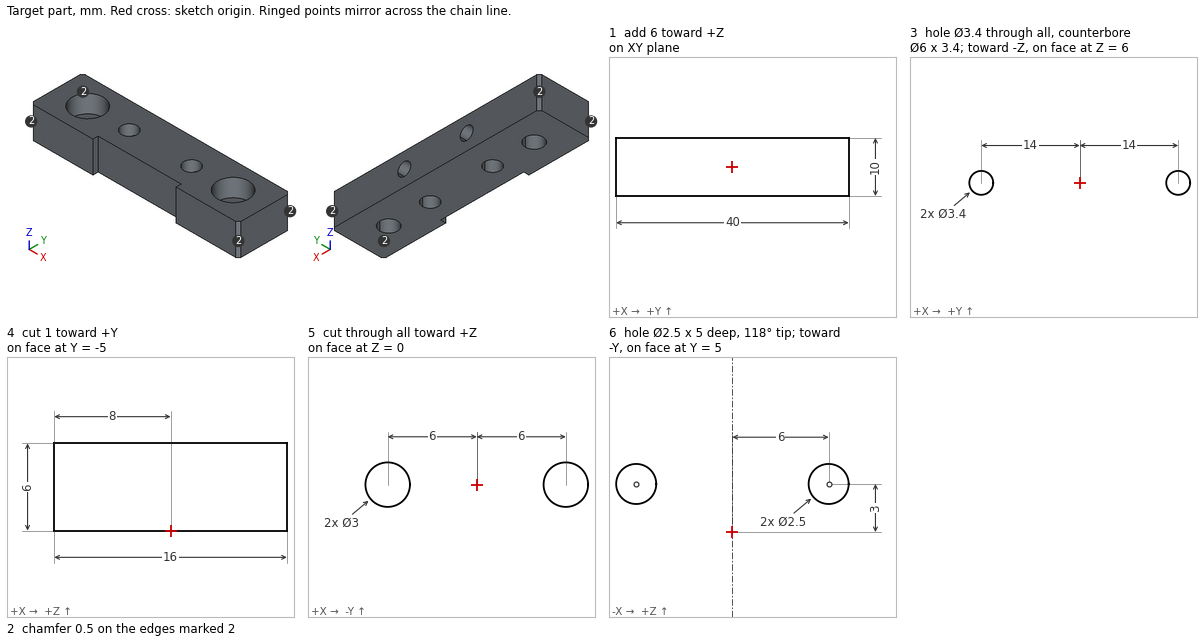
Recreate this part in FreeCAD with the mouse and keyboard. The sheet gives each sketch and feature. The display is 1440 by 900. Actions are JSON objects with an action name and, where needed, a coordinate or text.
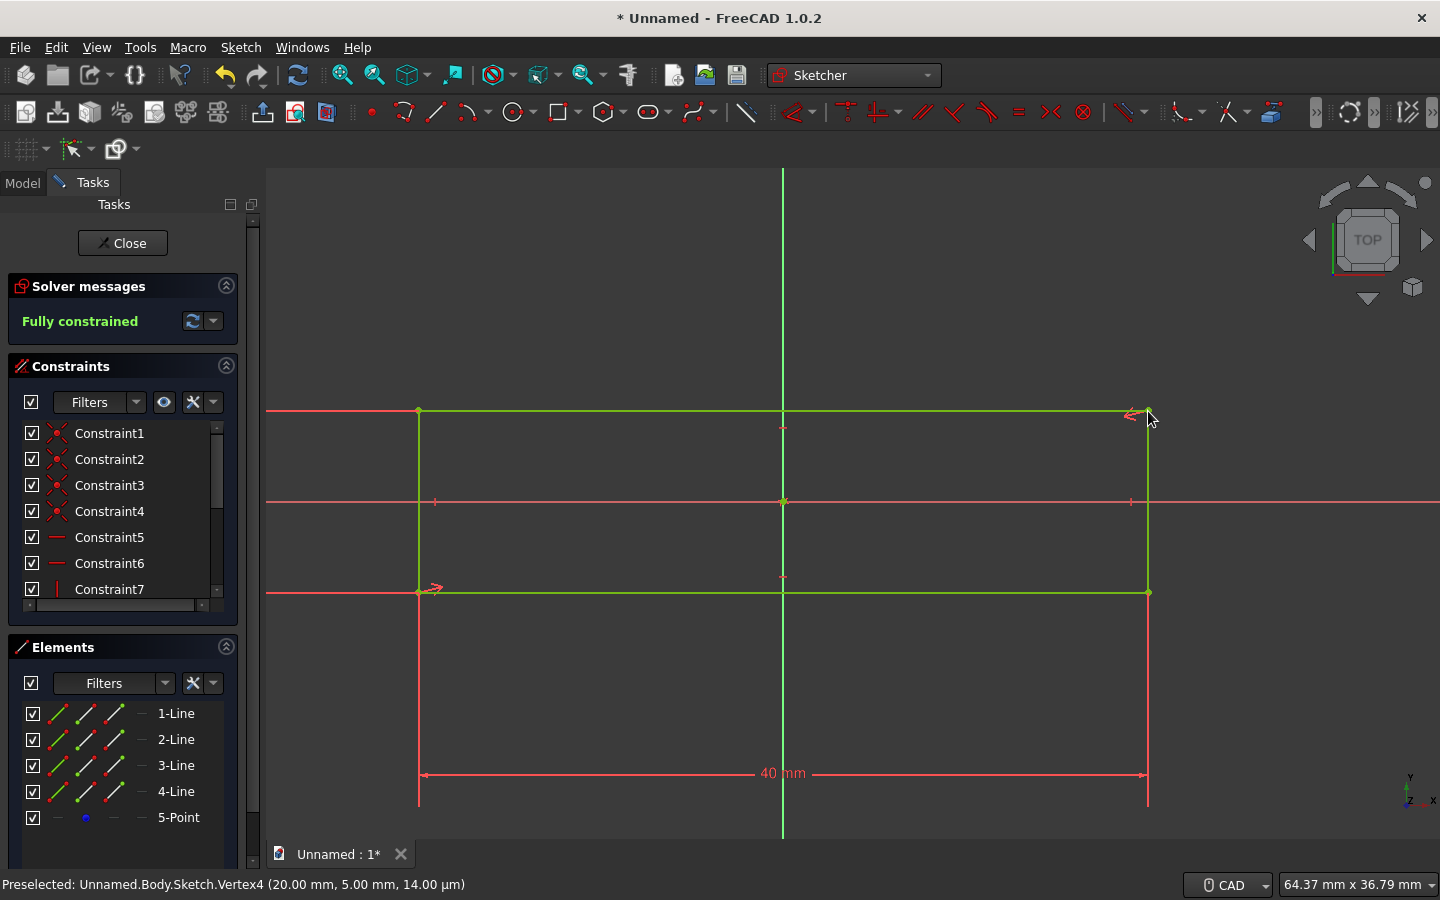
{"action": "left_click", "coordinate": [123, 243]}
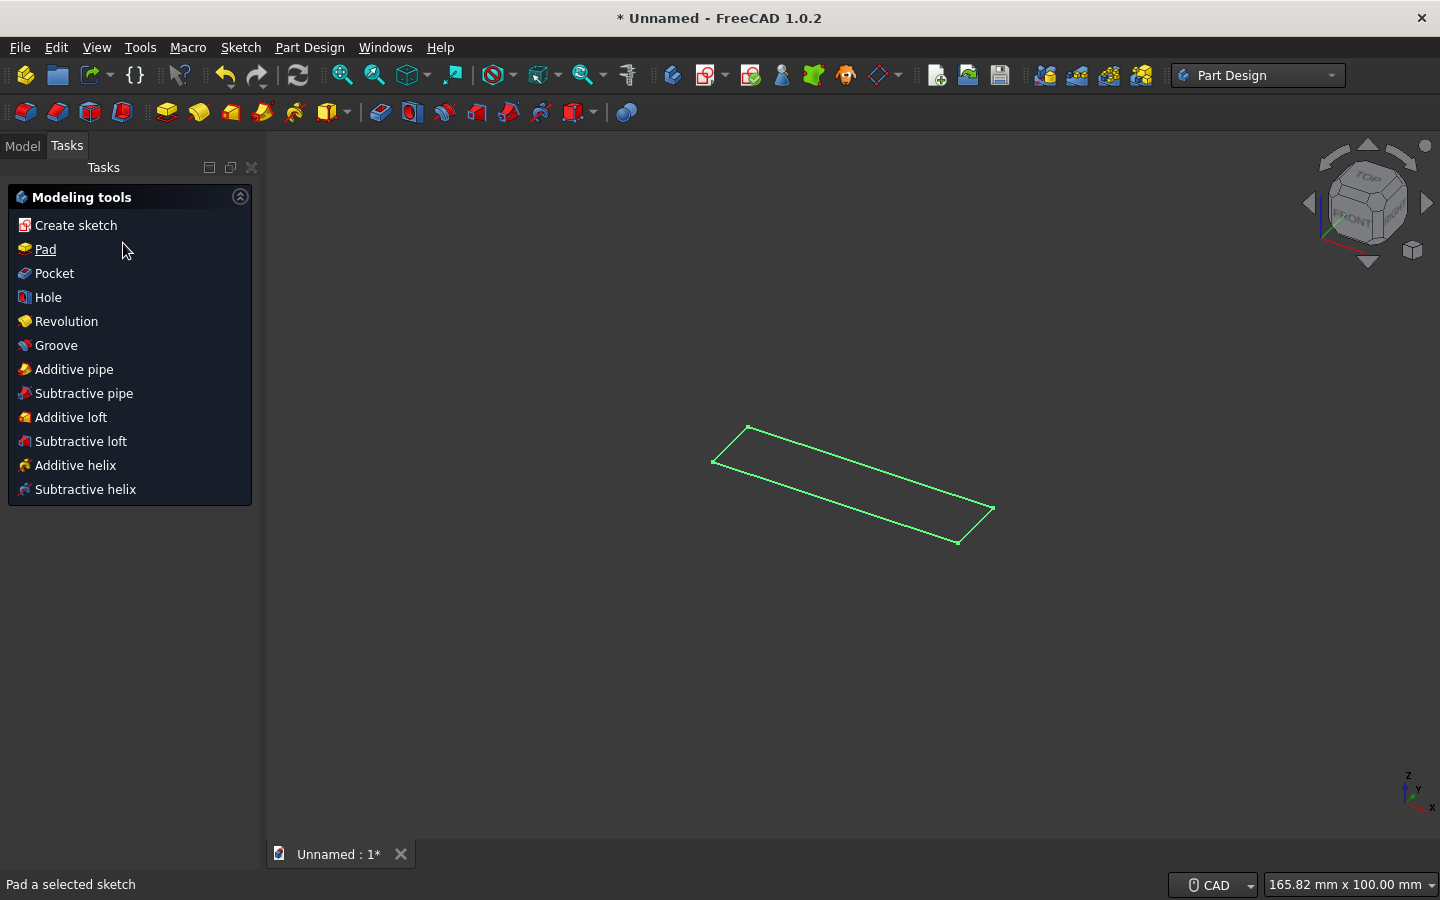
{"action": "left_click", "coordinate": [168, 112]}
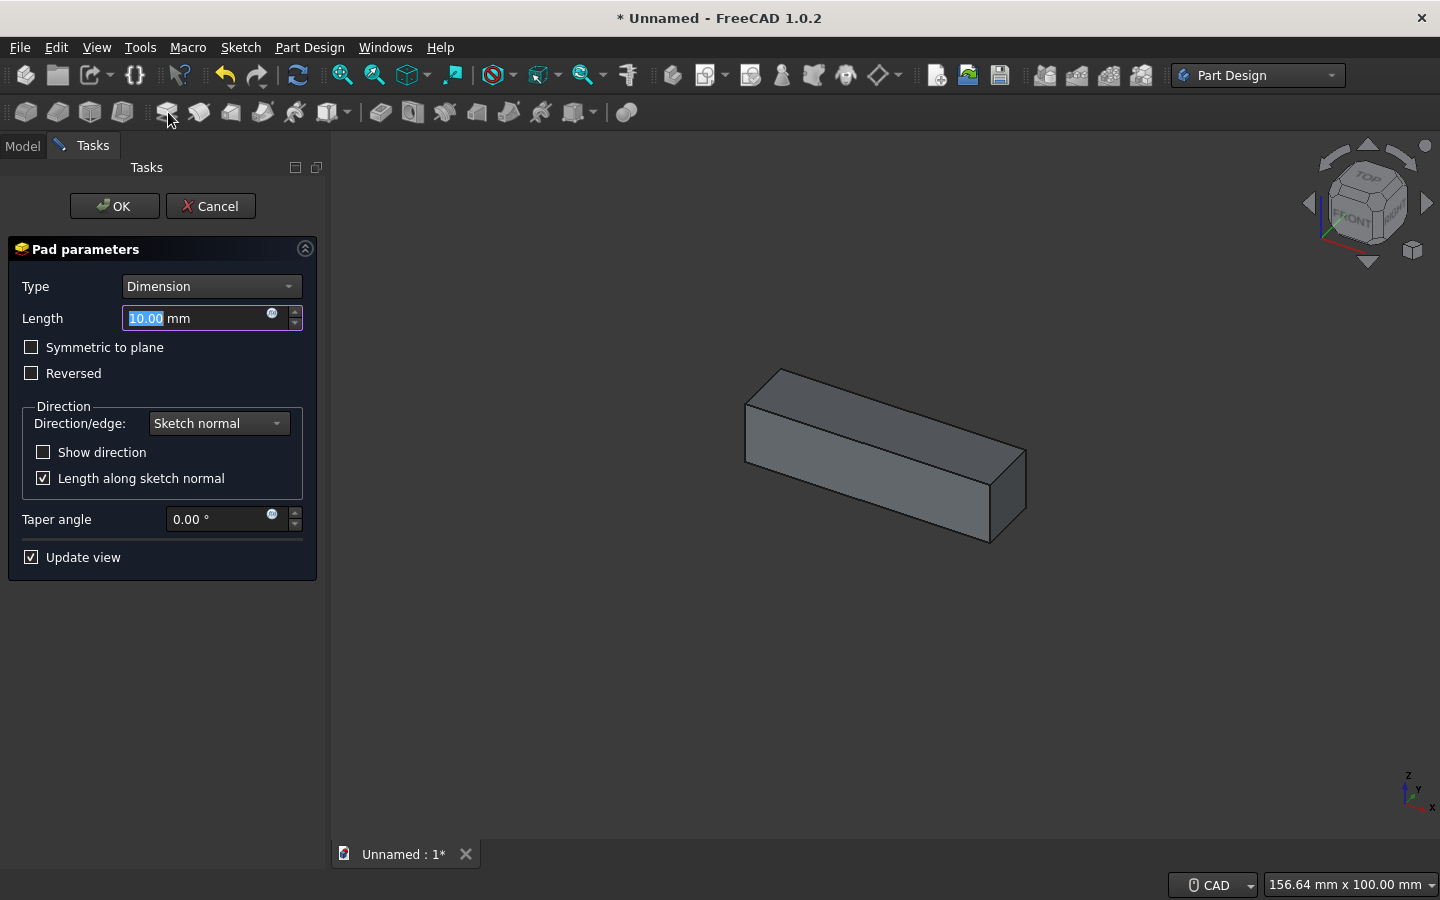
{"action": "type", "text": "6"}
{"action": "key", "text": "Tab"}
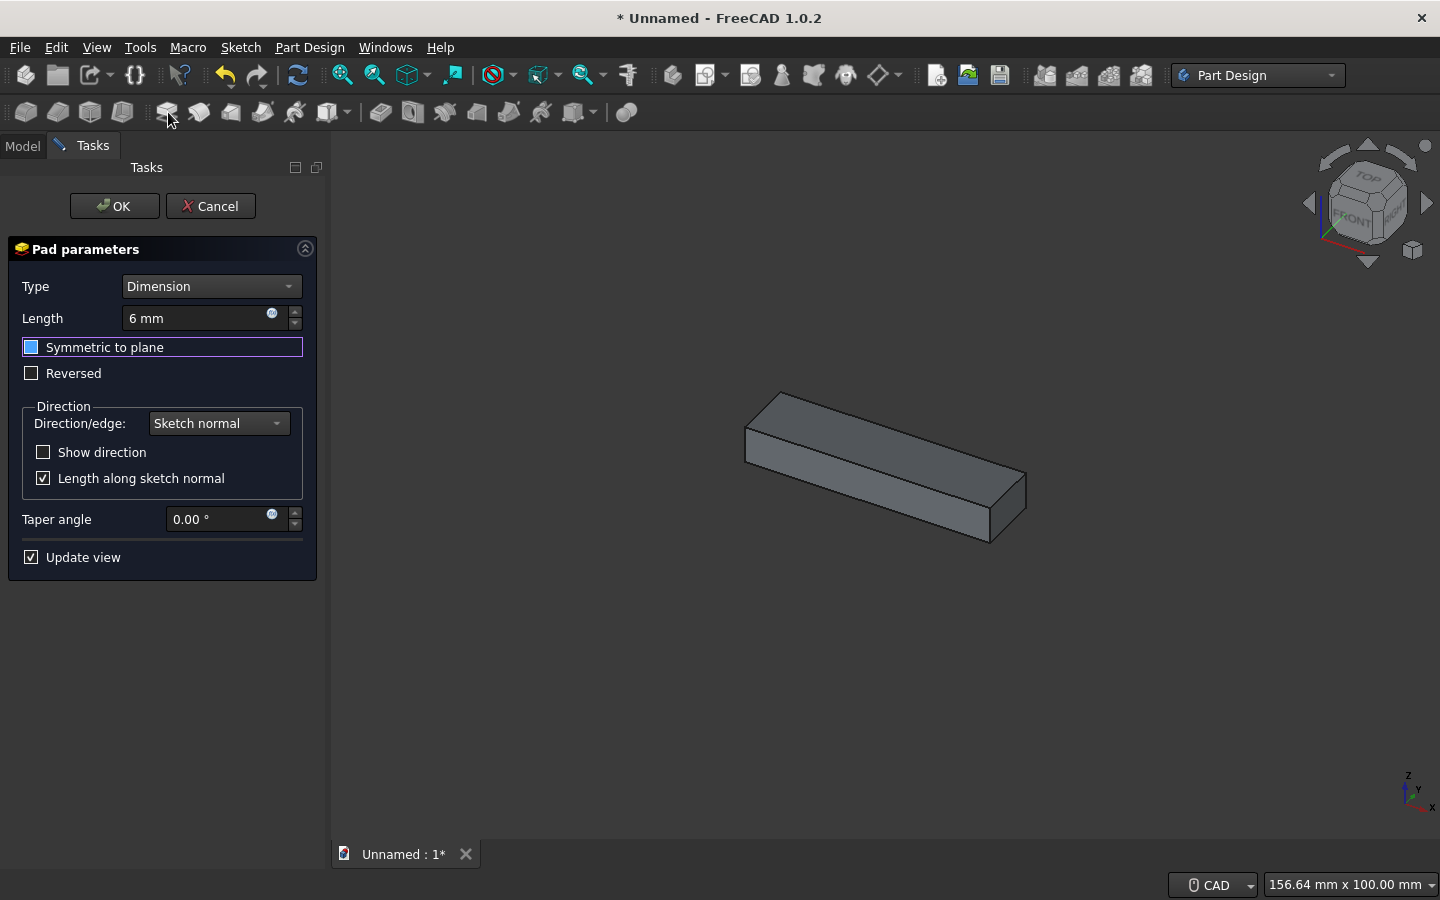
{"action": "left_click", "coordinate": [115, 206]}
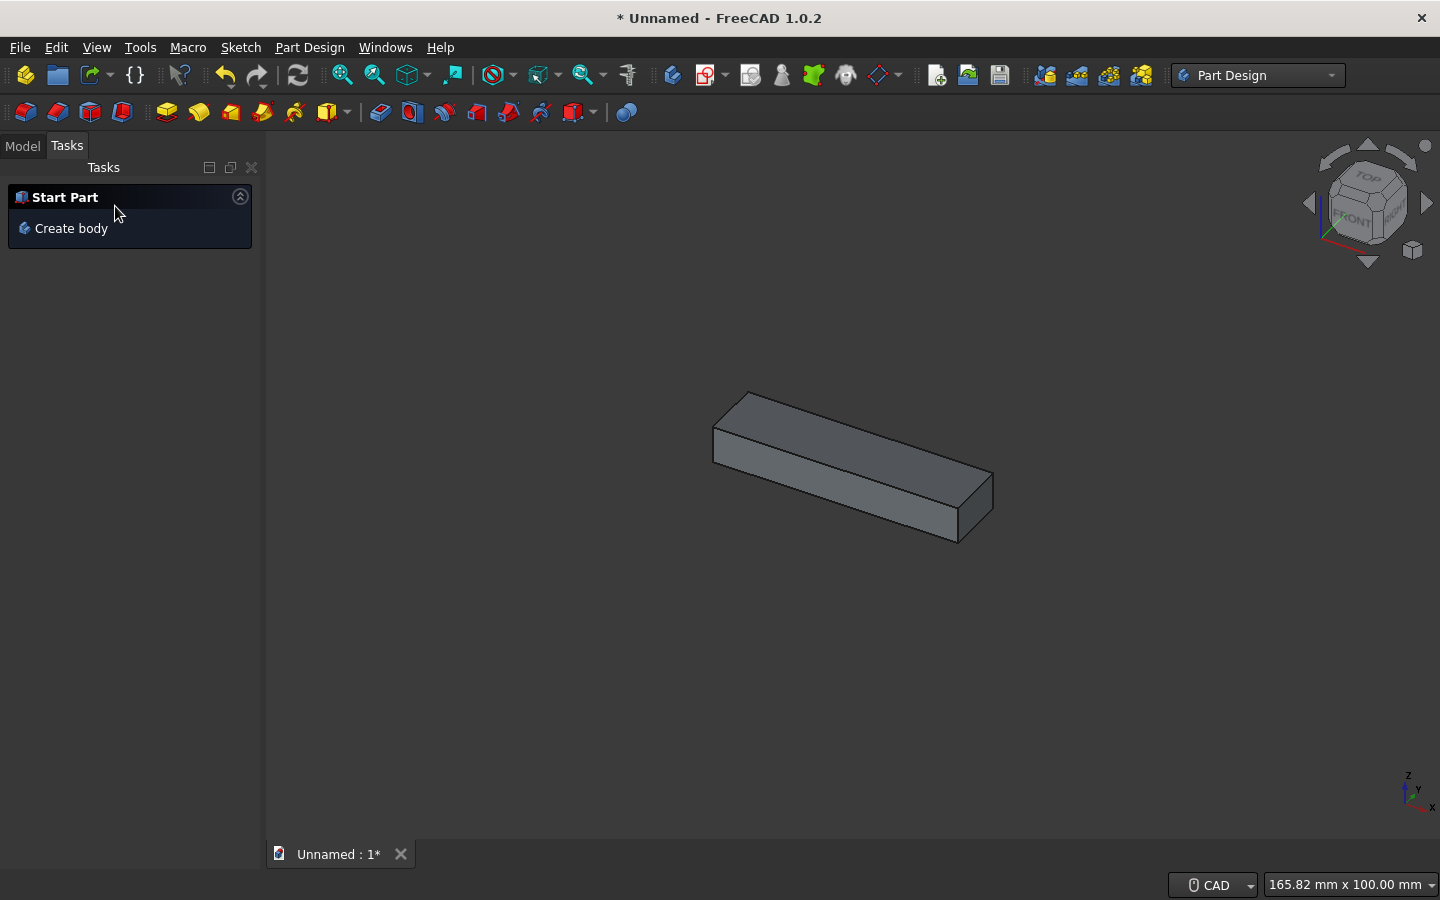
{"action": "left_click", "coordinate": [344, 76]}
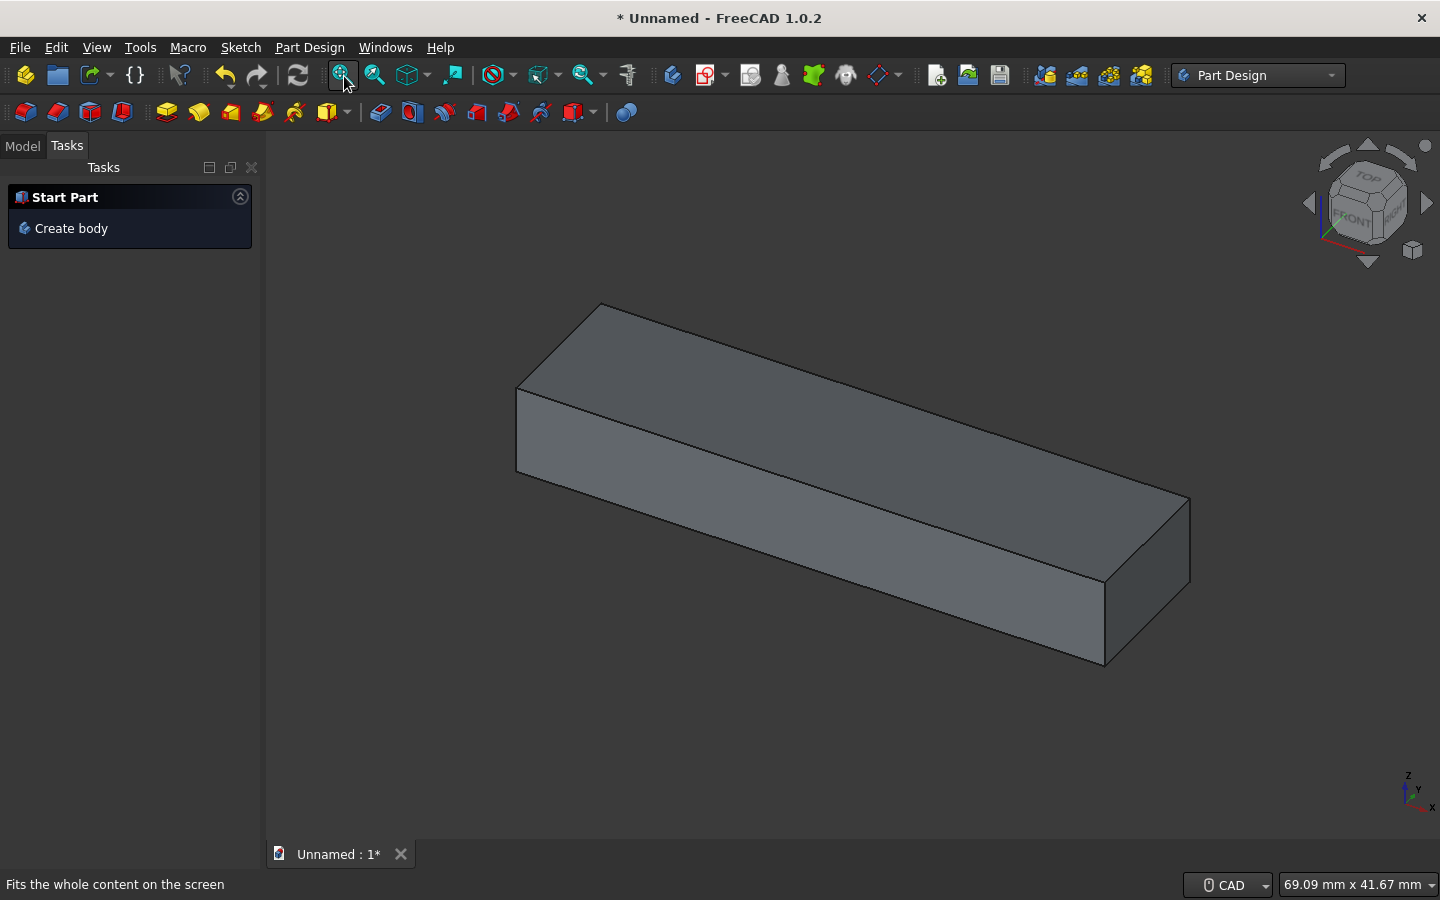
{"action": "left_click", "coordinate": [1105, 624]}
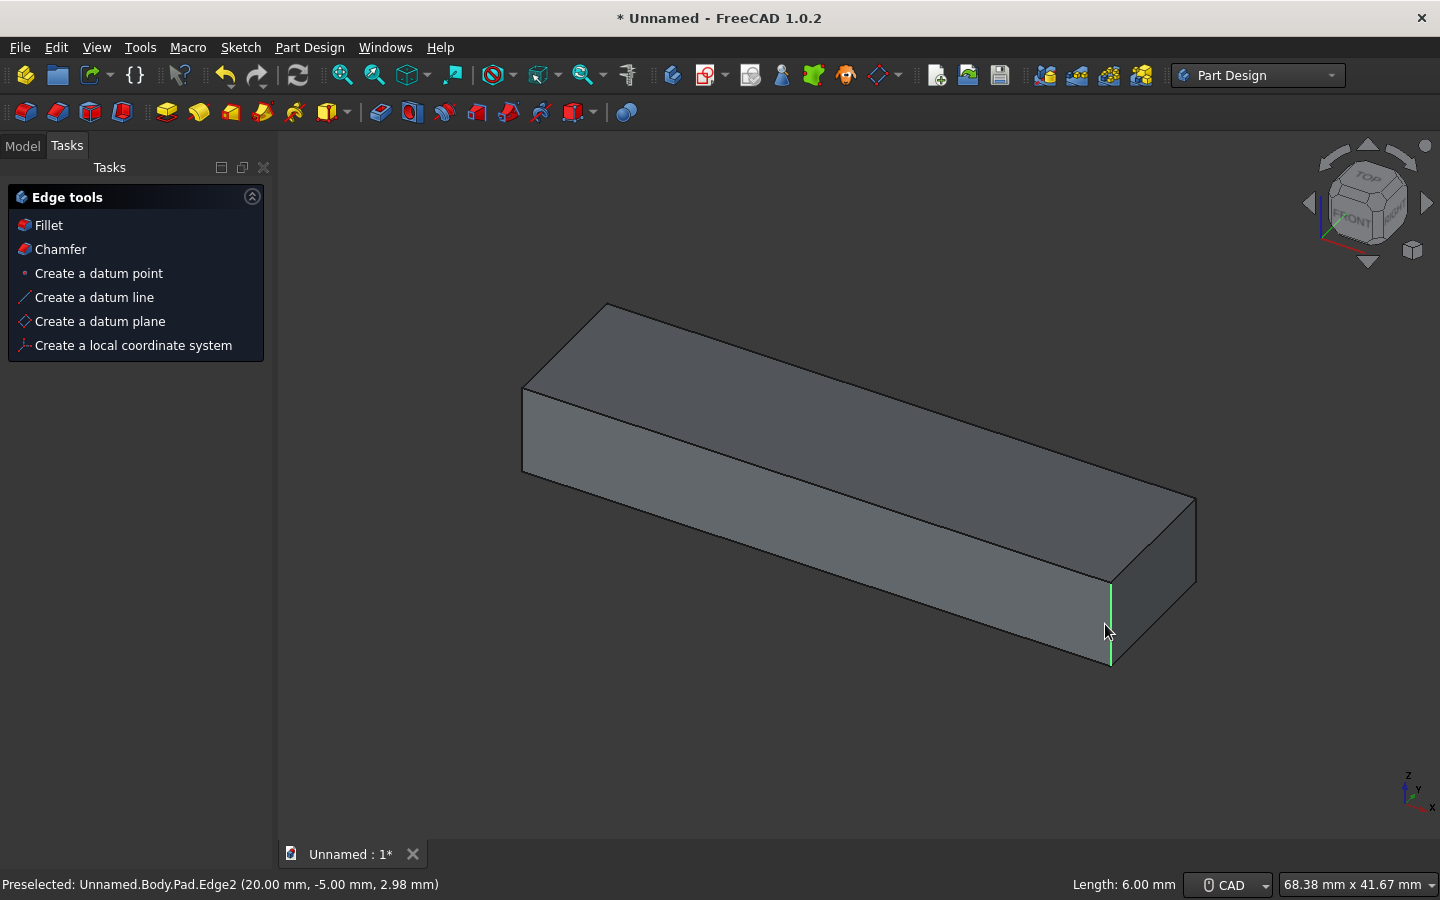
{"action": "key", "text": "0"}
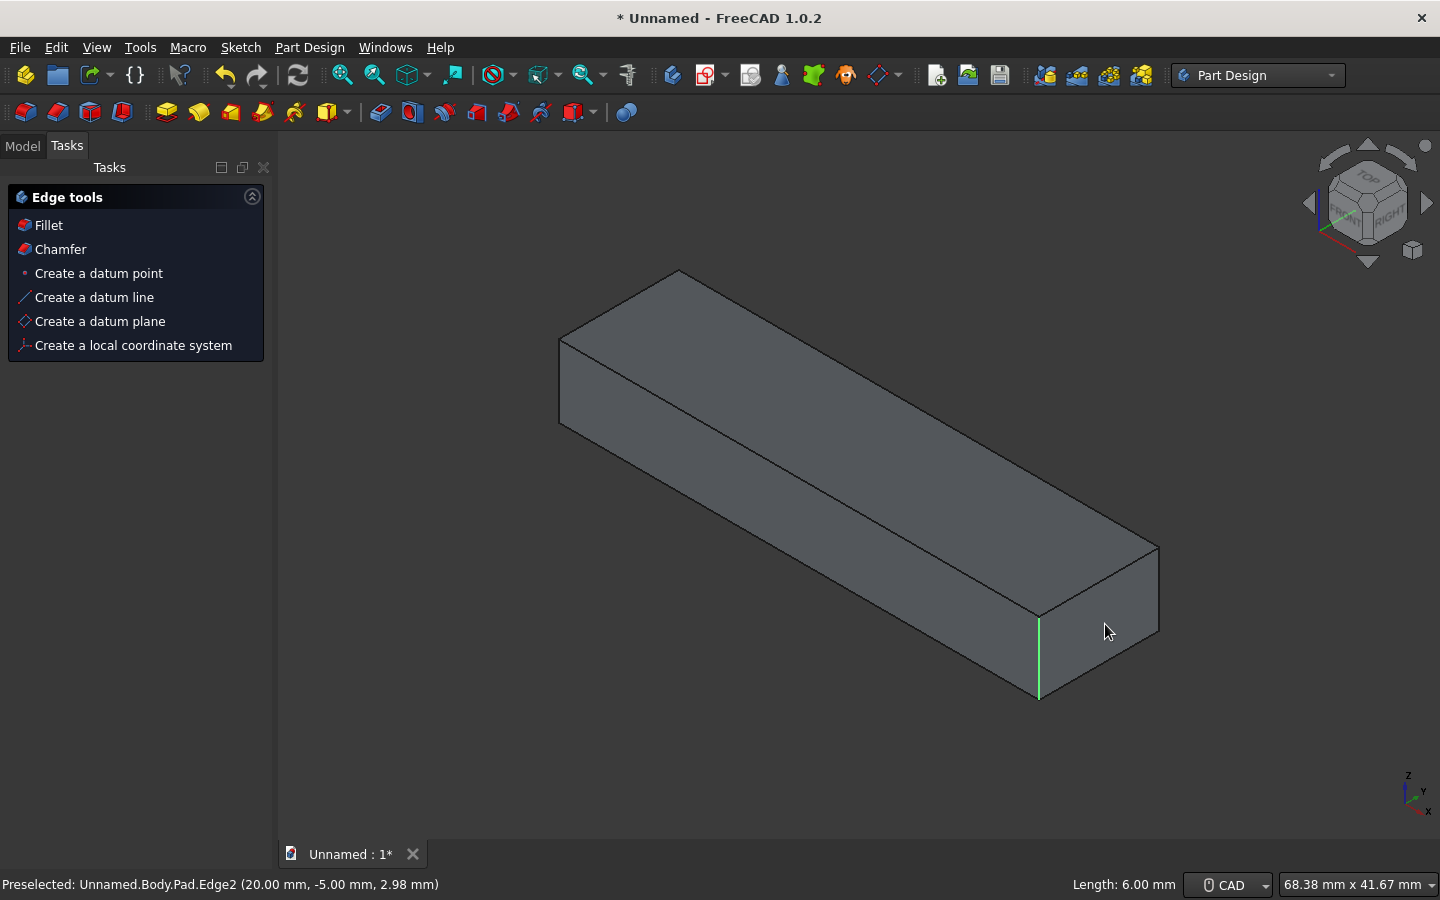
{"action": "key", "text": "2"}